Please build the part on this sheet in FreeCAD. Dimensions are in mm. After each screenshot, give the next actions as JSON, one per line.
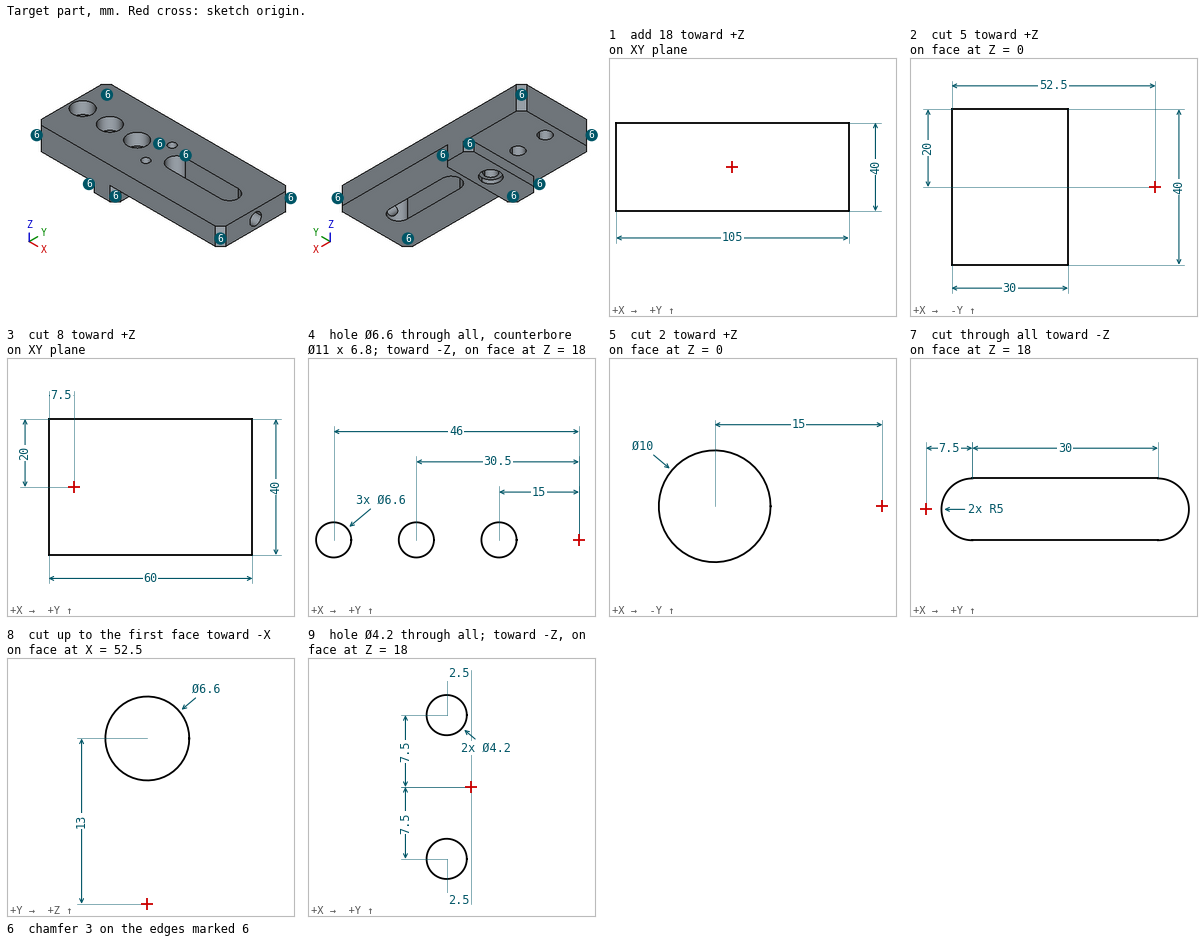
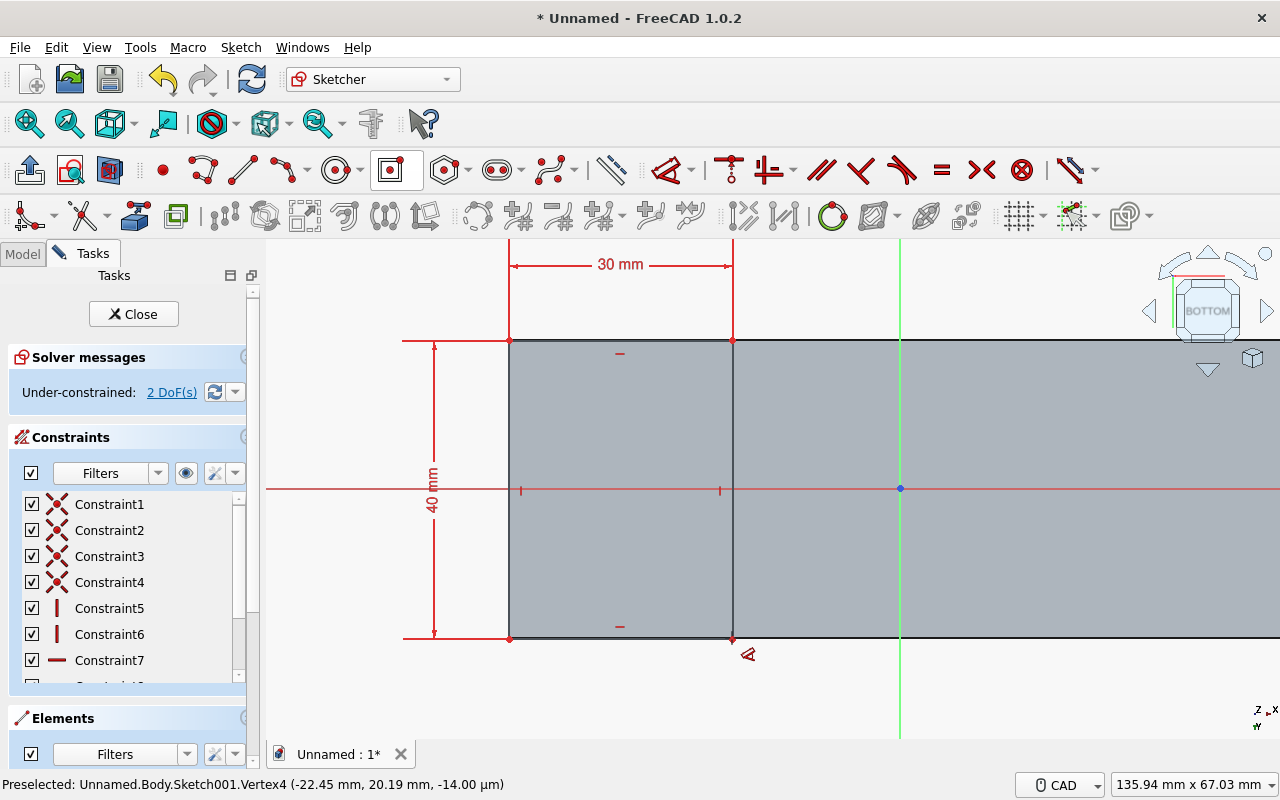
{"action": "left_click", "coordinate": [509, 341]}
{"action": "left_click", "coordinate": [934, 415]}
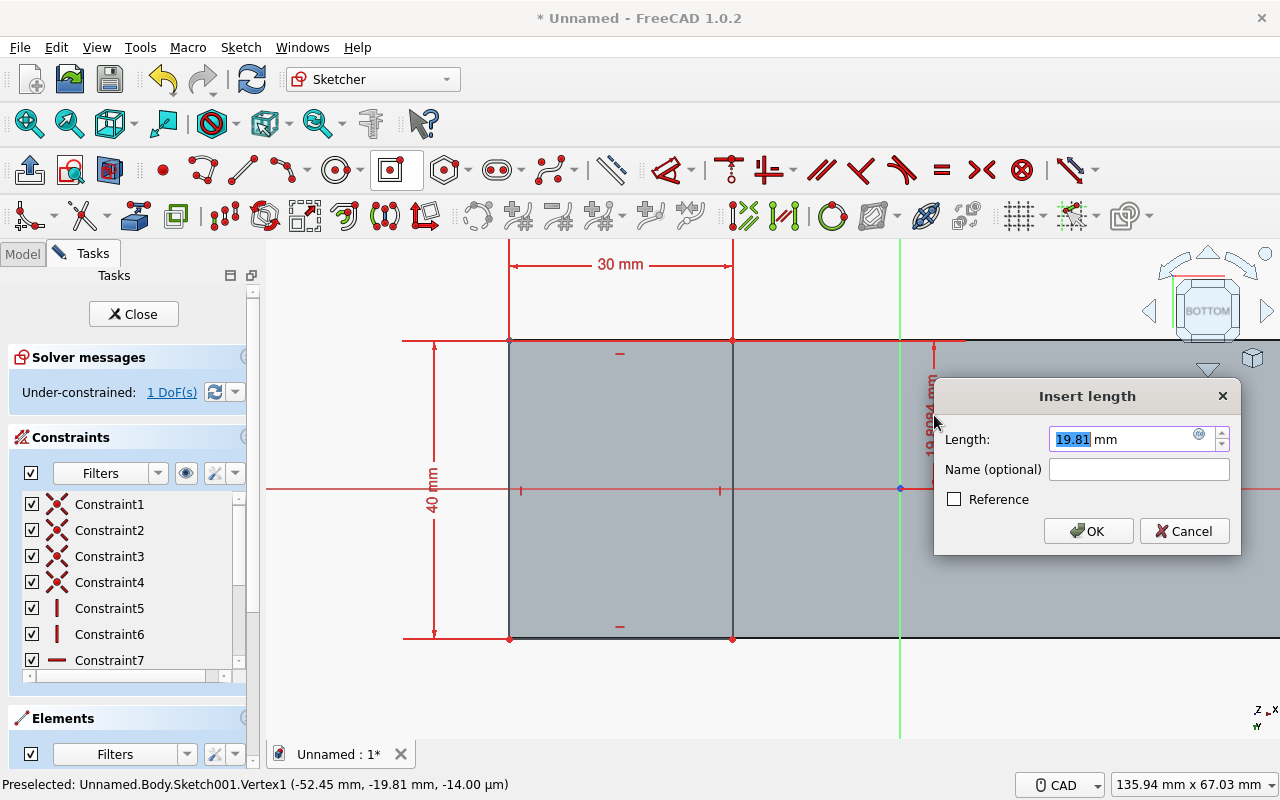
{"action": "type", "text": "20"}
{"action": "key", "text": "Return"}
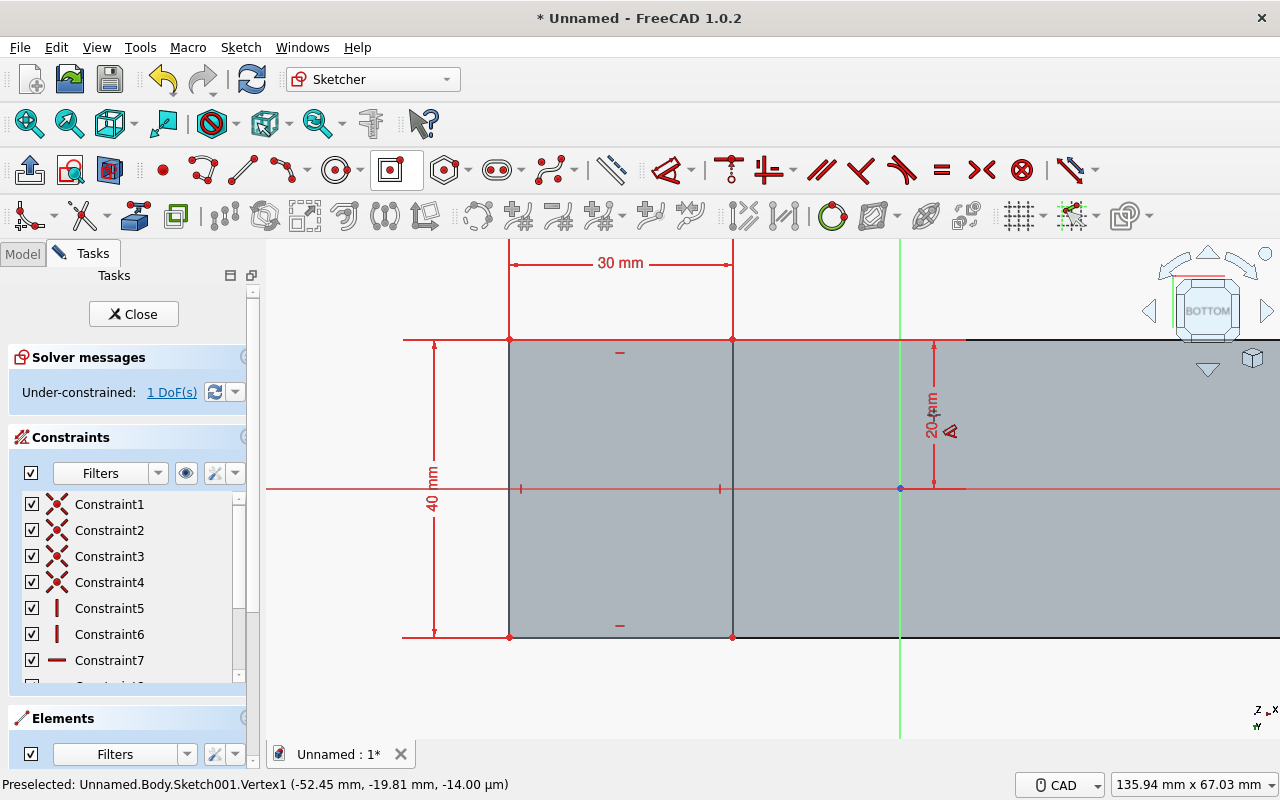
{"action": "left_click", "coordinate": [509, 340]}
{"action": "left_click", "coordinate": [705, 306]}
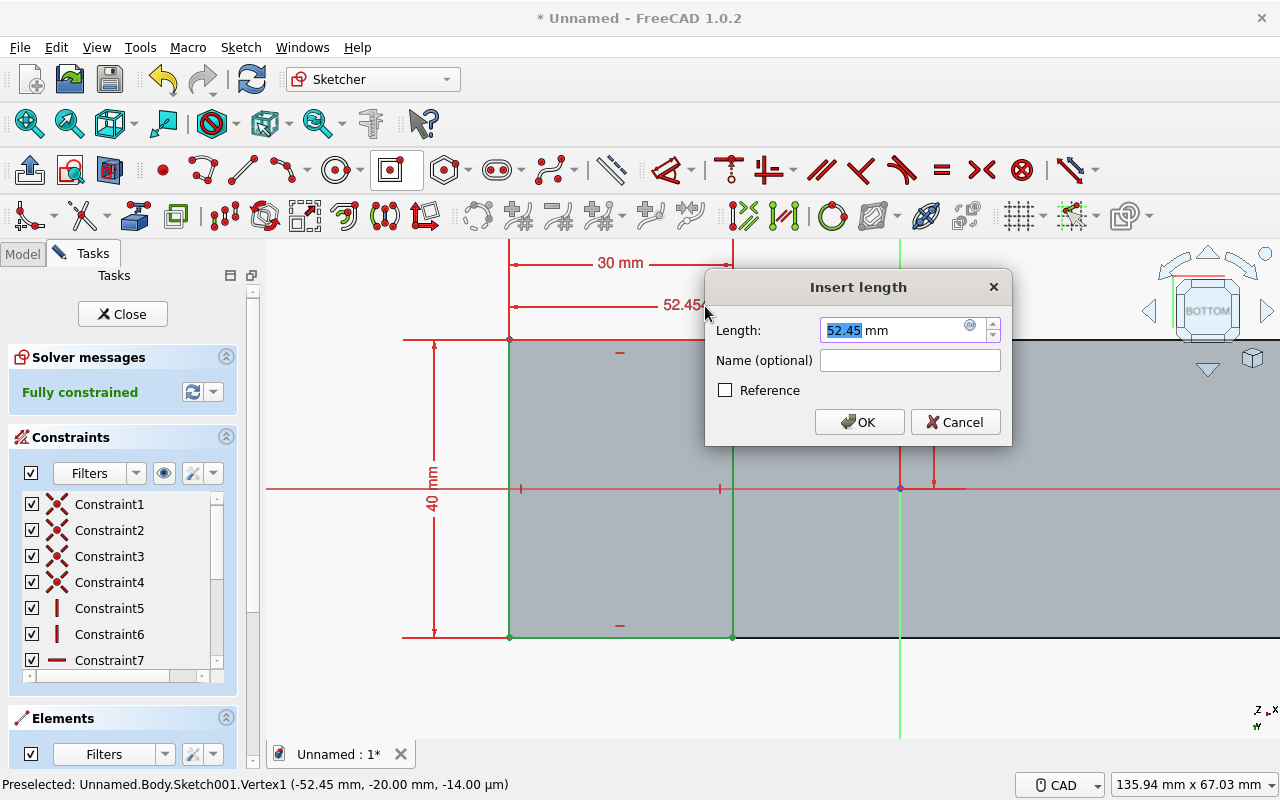
{"action": "type", "text": "52.5"}
{"action": "key", "text": "Return"}
{"action": "key", "text": "Escape"}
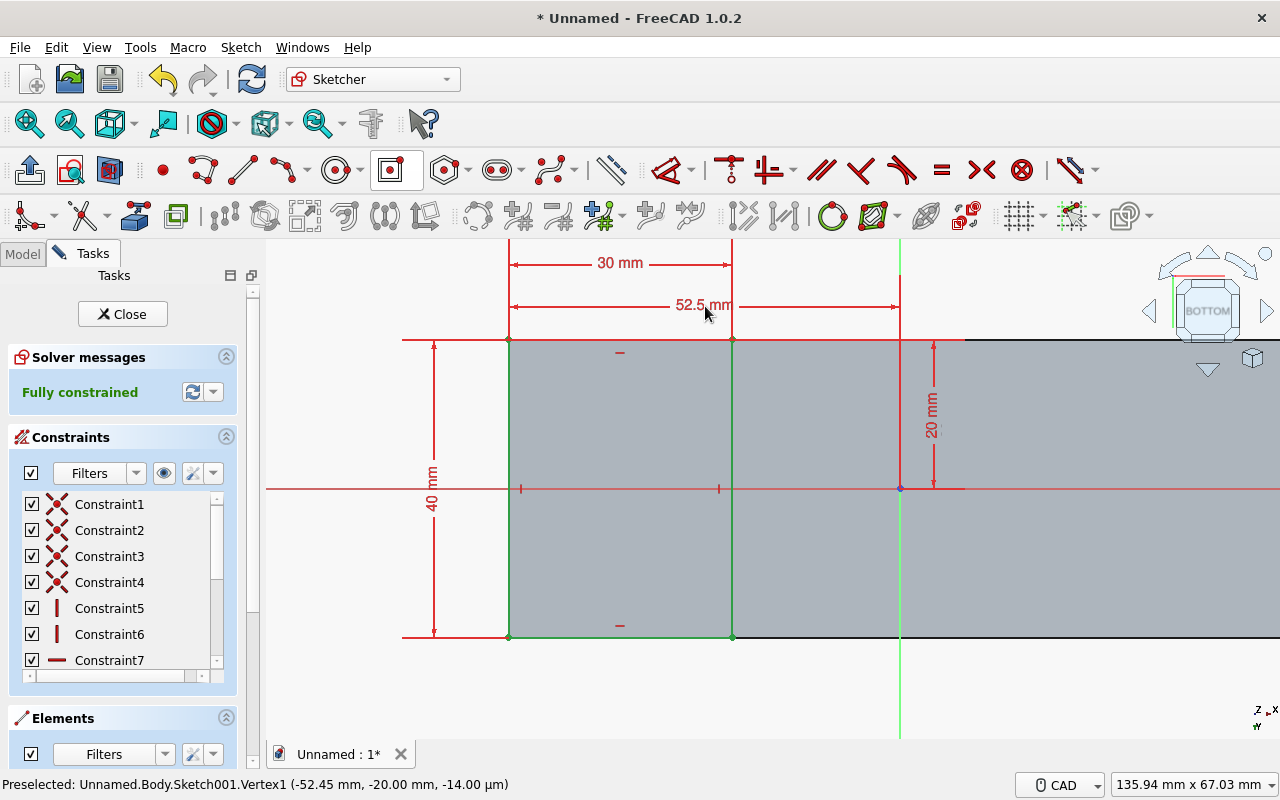
{"action": "left_click", "coordinate": [123, 314]}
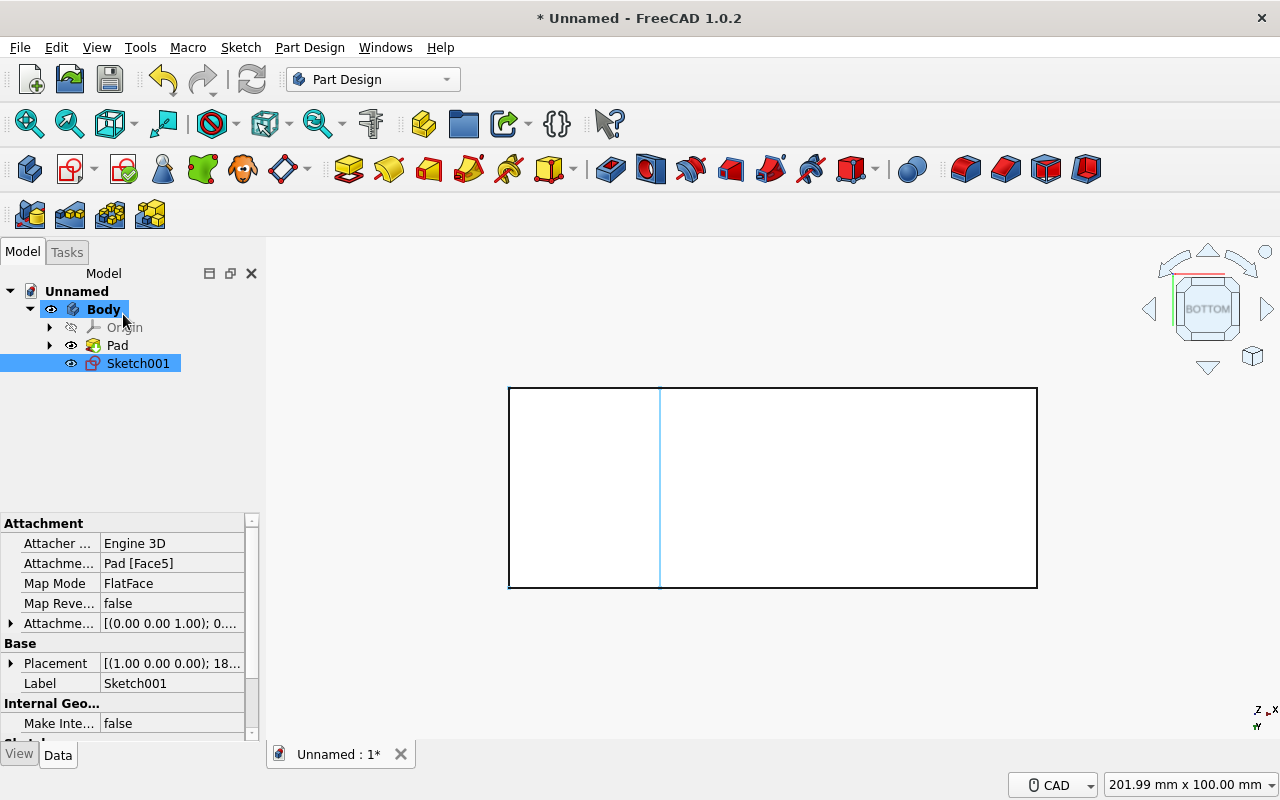
{"action": "left_click", "coordinate": [612, 170]}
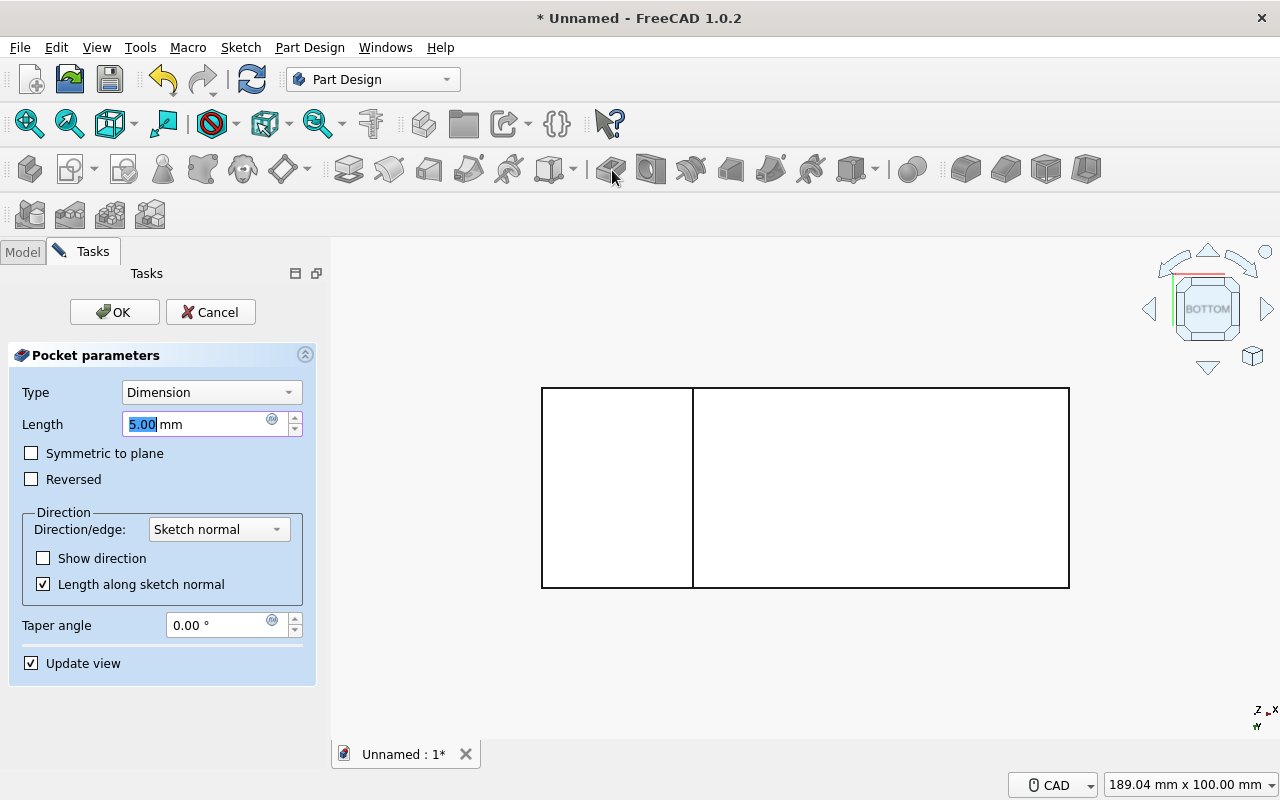
{"action": "type", "text": "5"}
{"action": "key", "text": "Tab"}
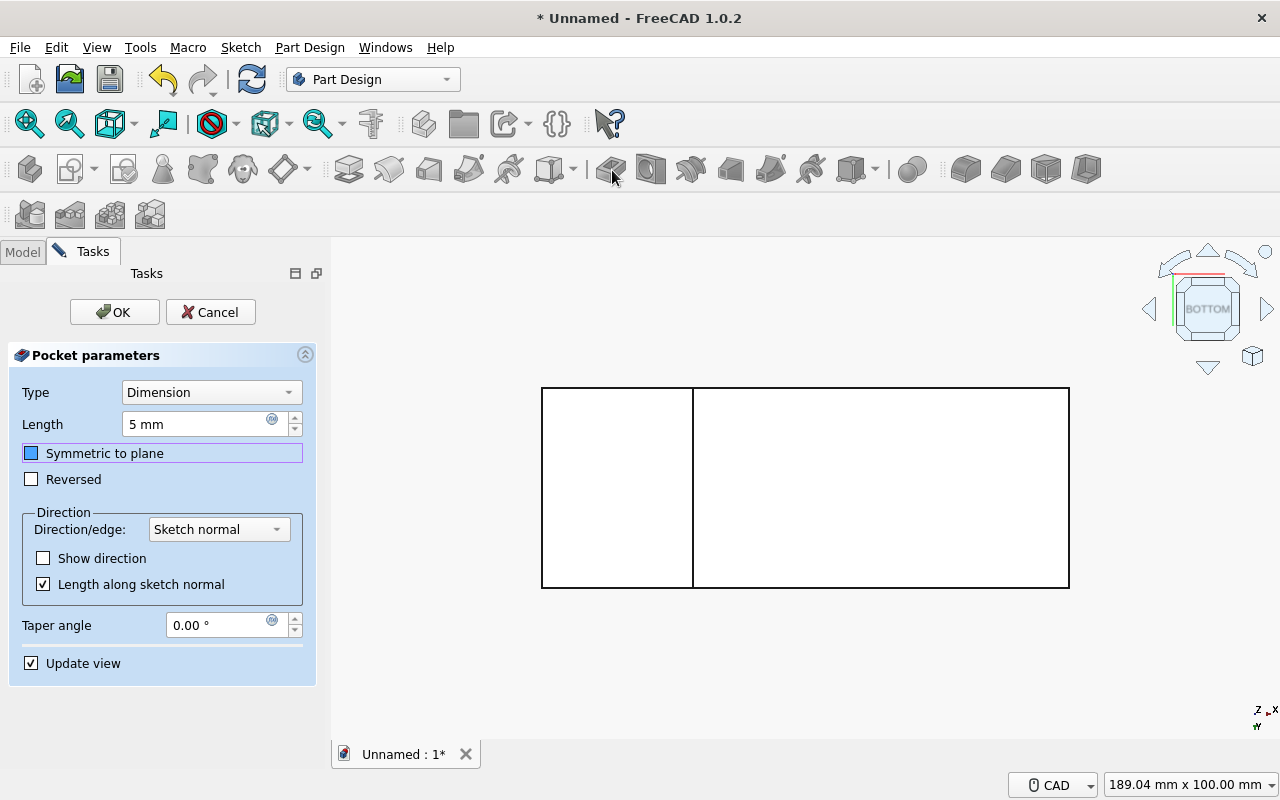
{"action": "left_click", "coordinate": [115, 312]}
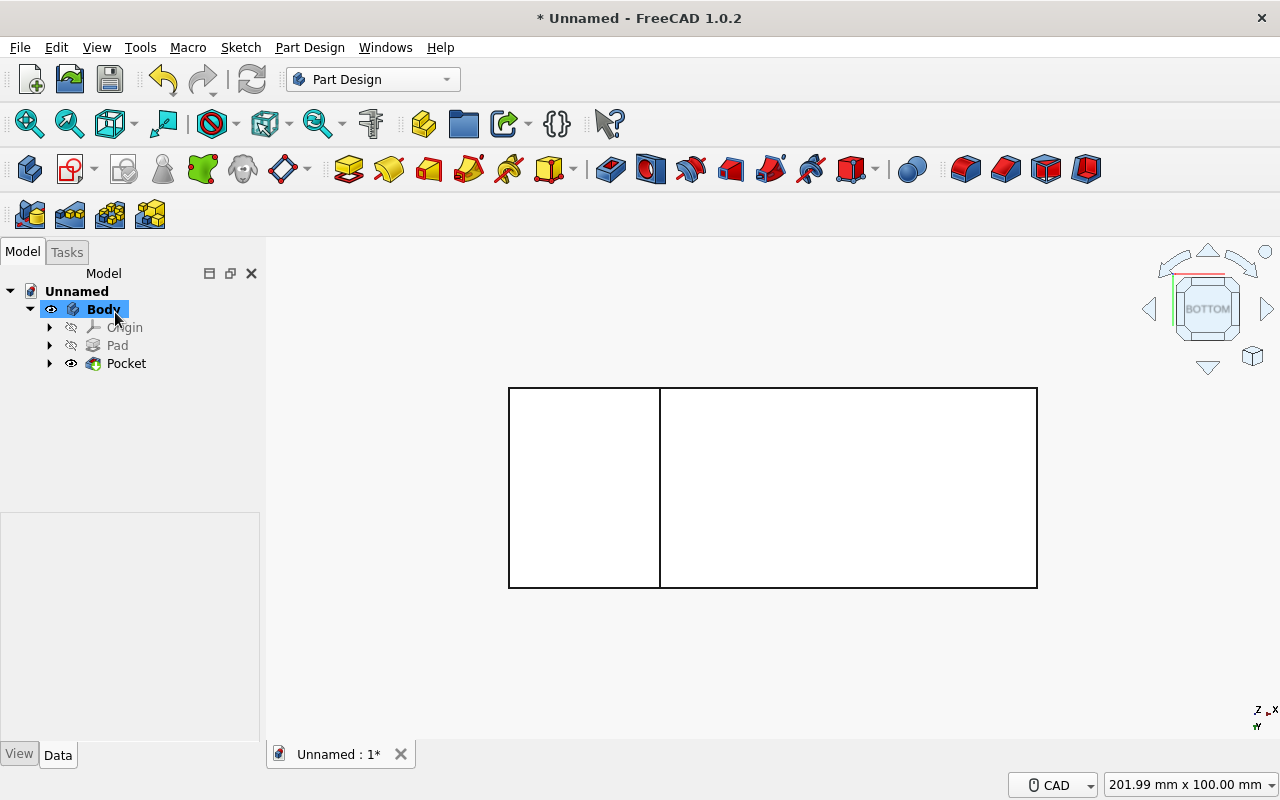
{"action": "left_click", "coordinate": [70, 170]}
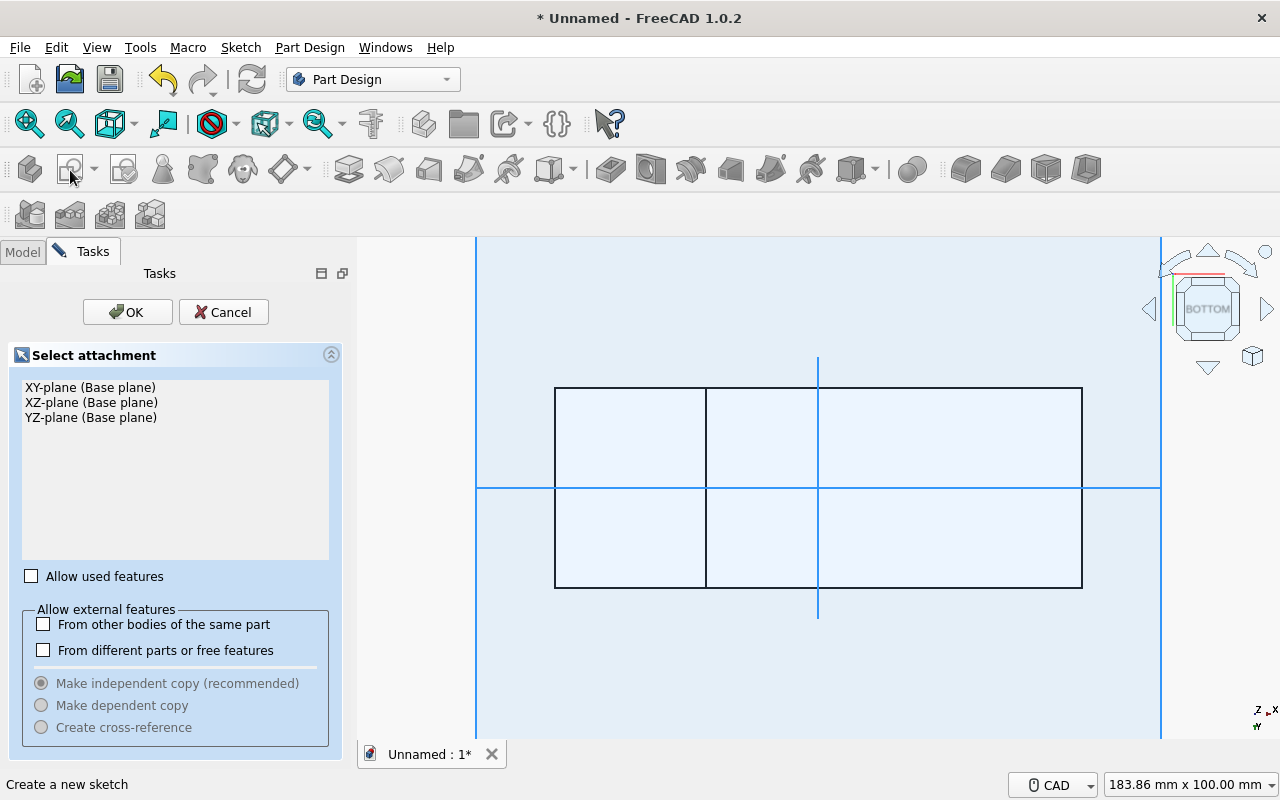
{"action": "left_click", "coordinate": [82, 388]}